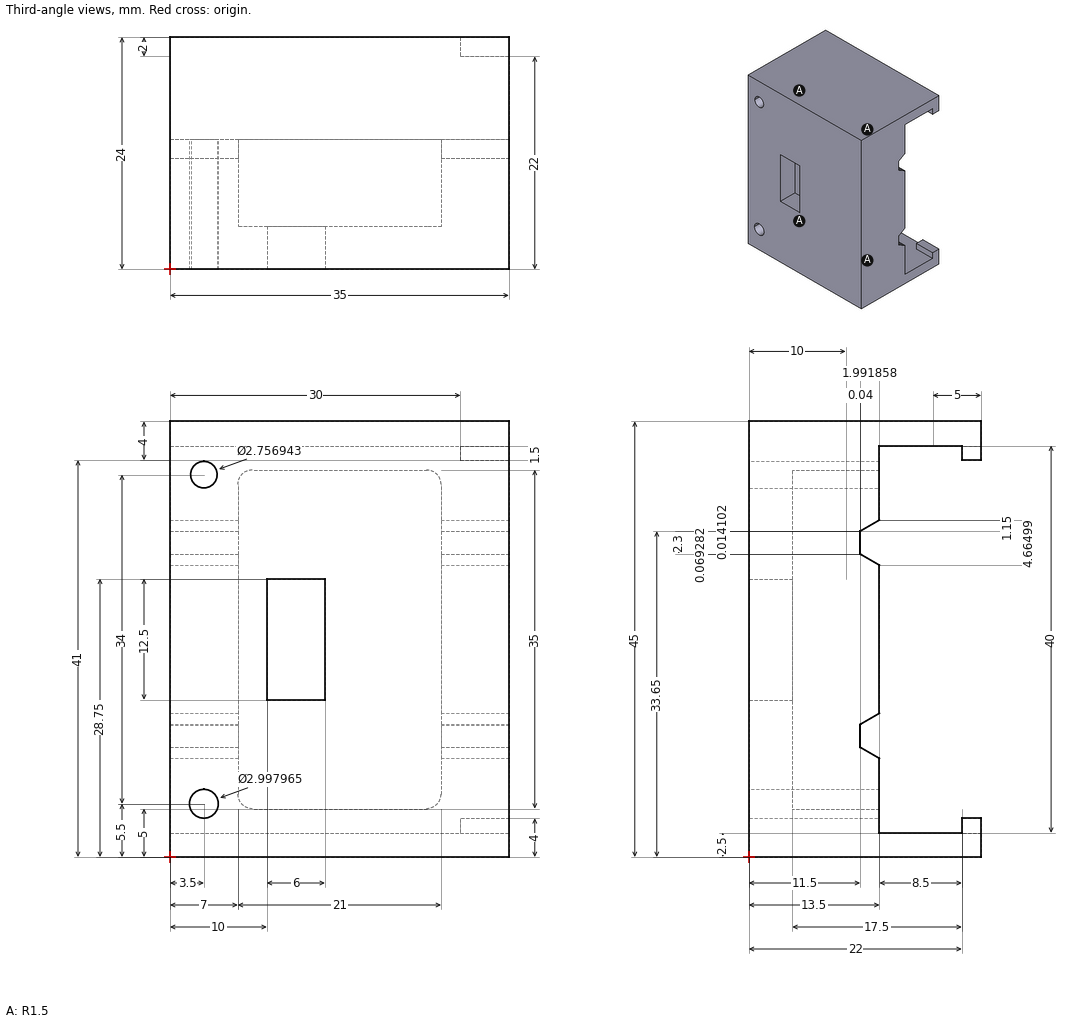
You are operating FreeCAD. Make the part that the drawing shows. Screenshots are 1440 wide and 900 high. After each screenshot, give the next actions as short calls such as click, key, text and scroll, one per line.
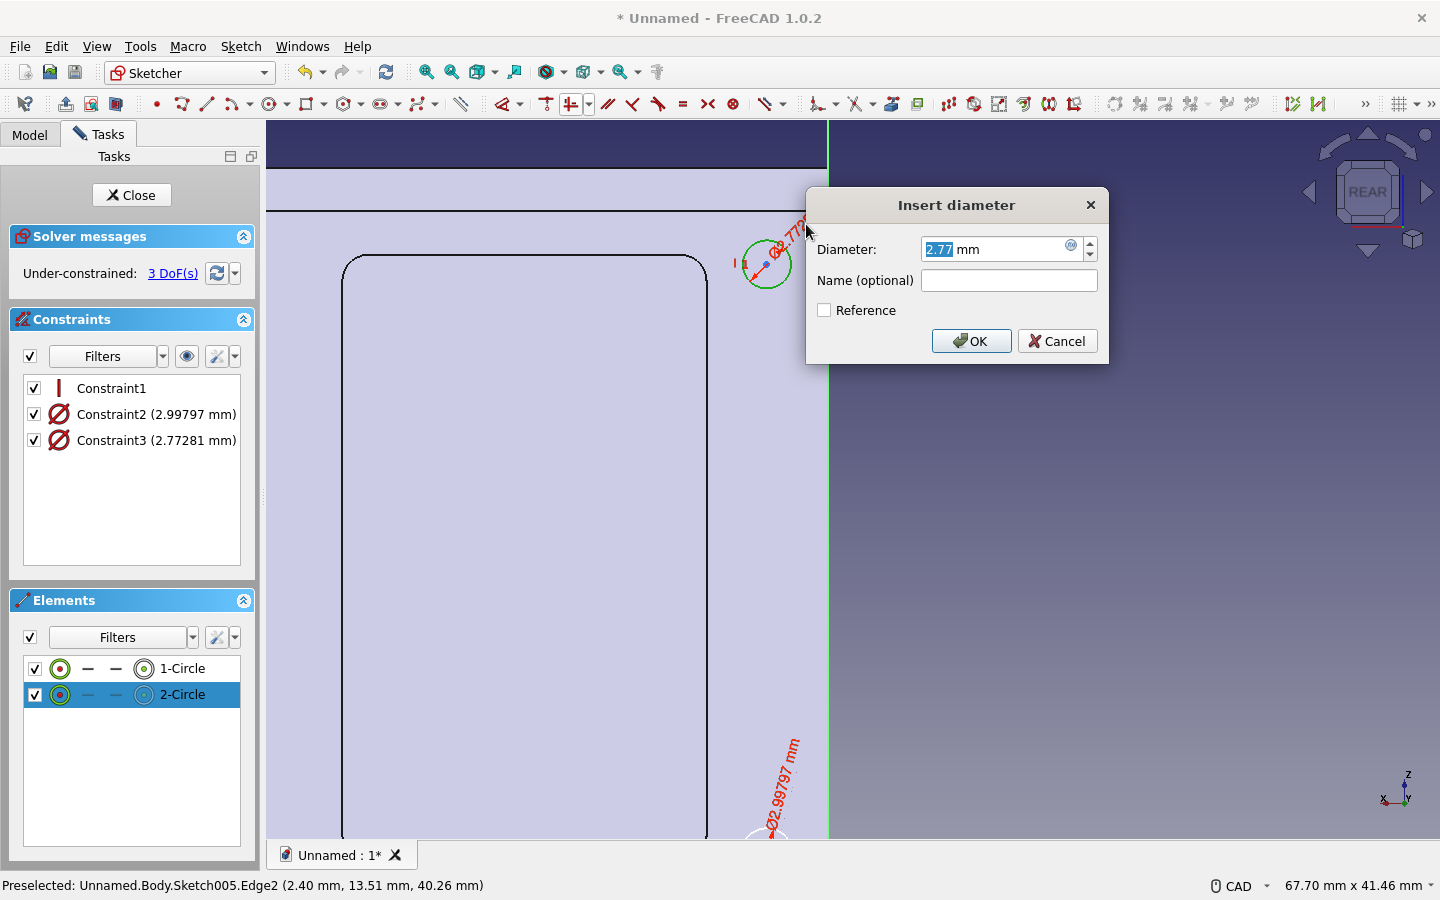
text(2.756943)
key(Return)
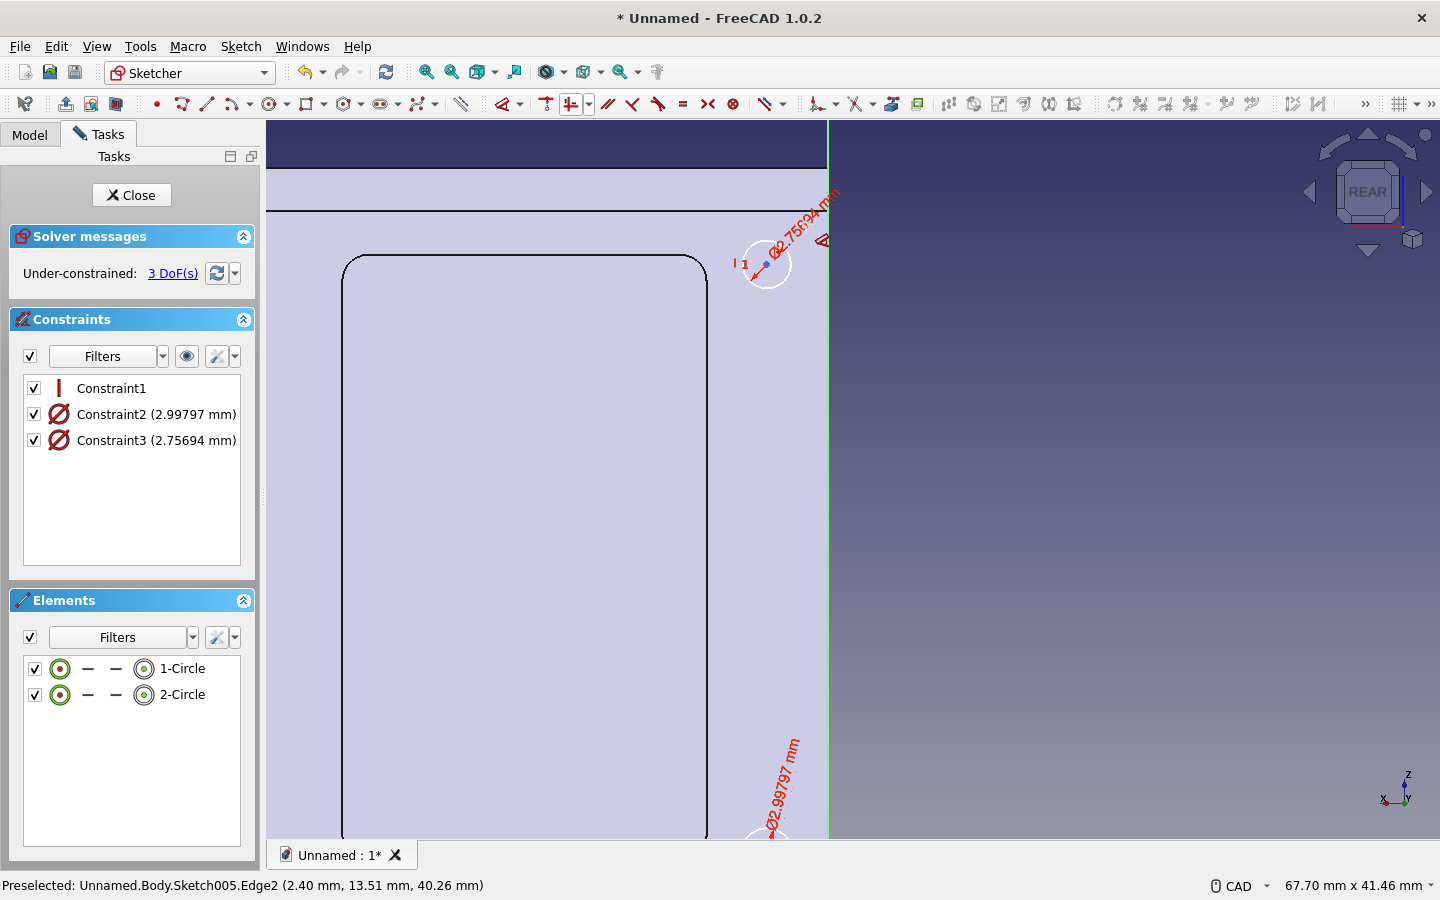
scroll(784, 247, down, 2)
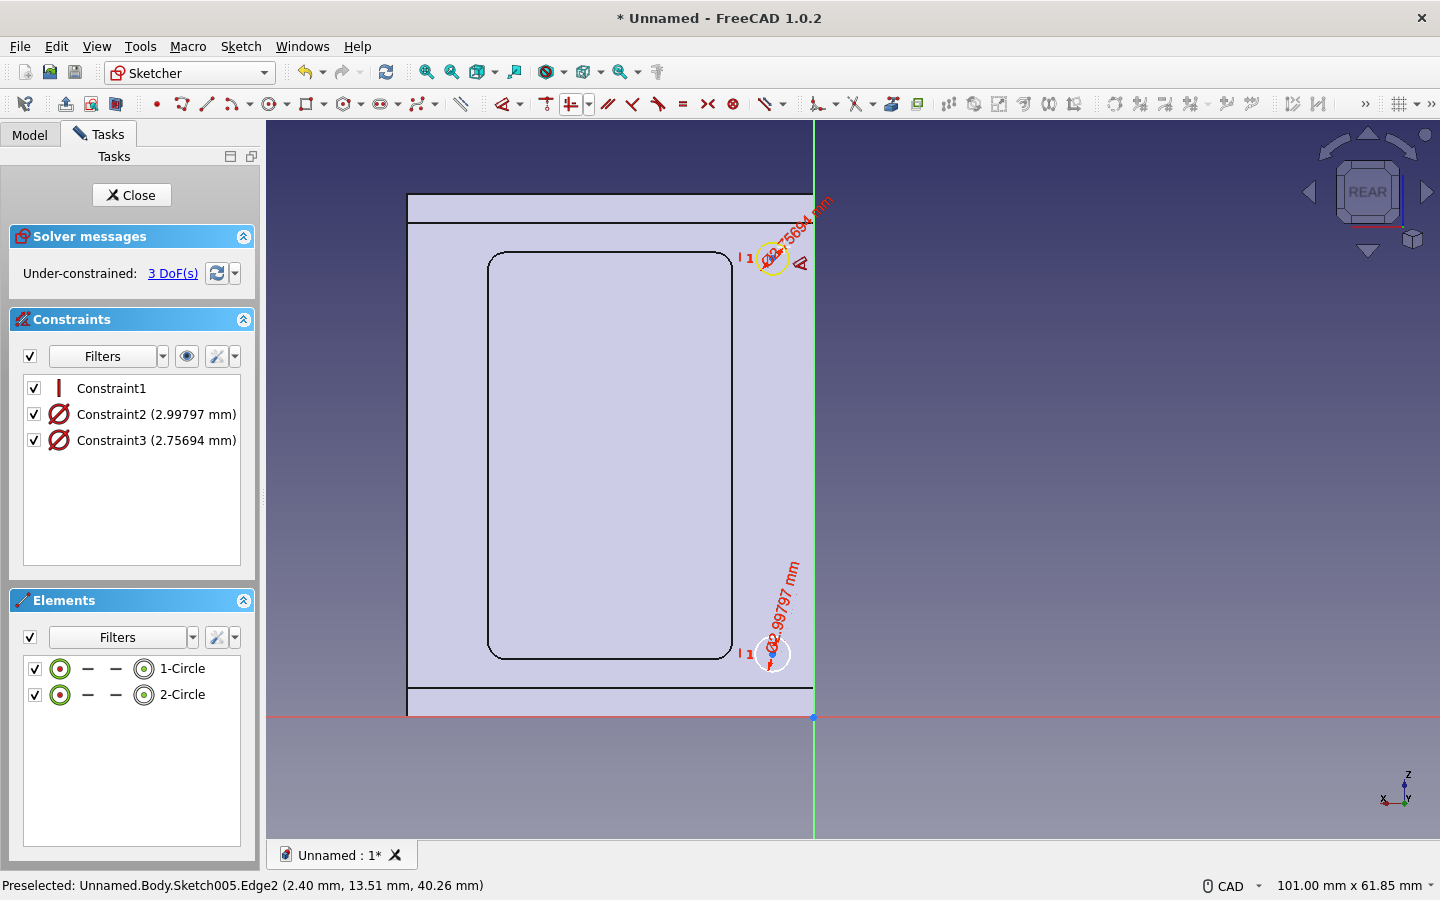
click(773, 654)
click(793, 751)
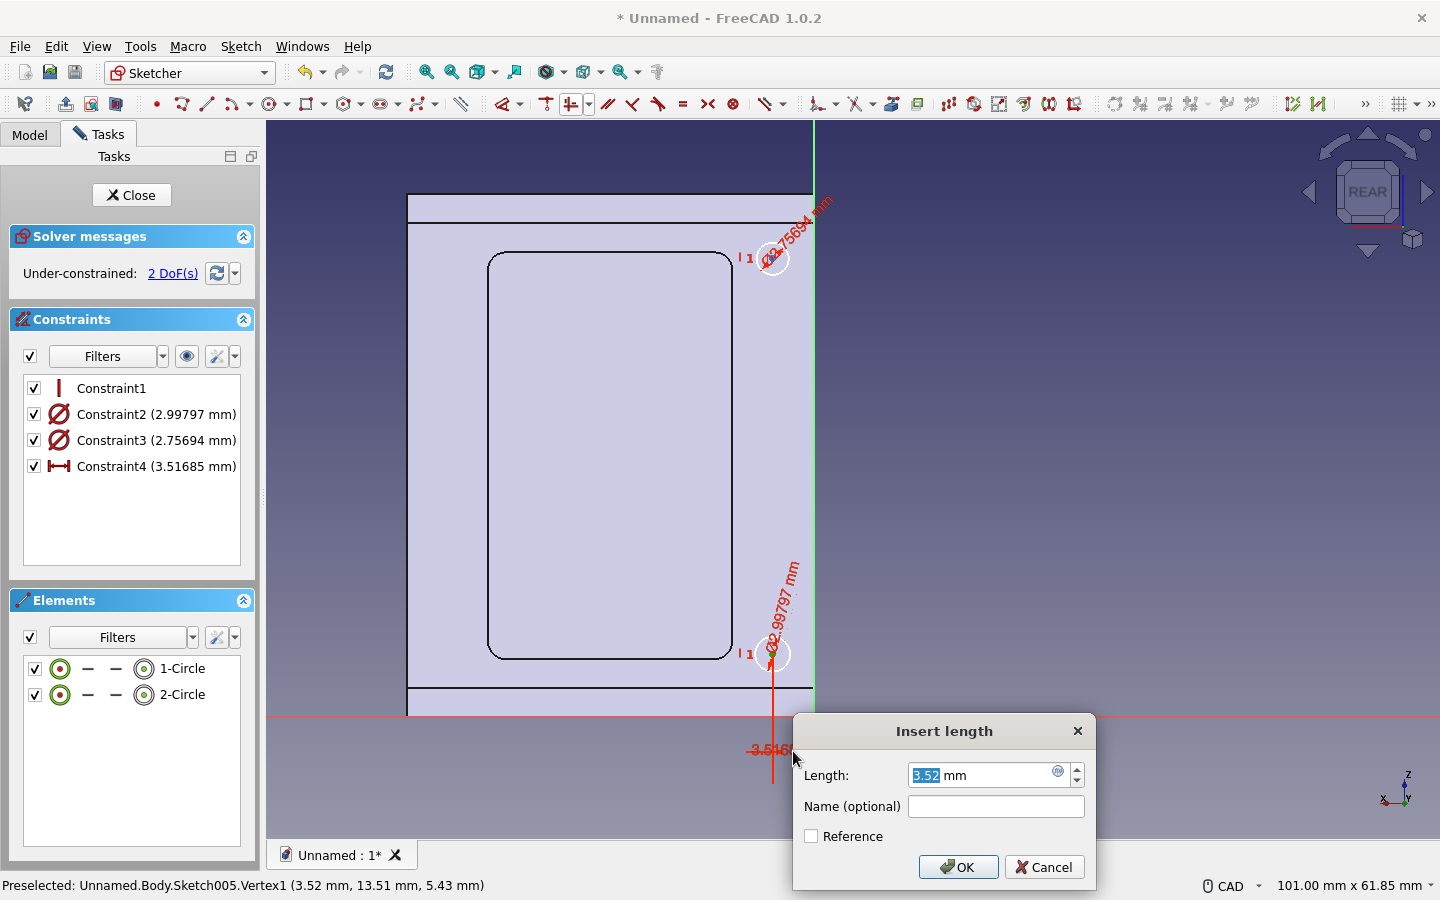
text(3.5)
key(Return)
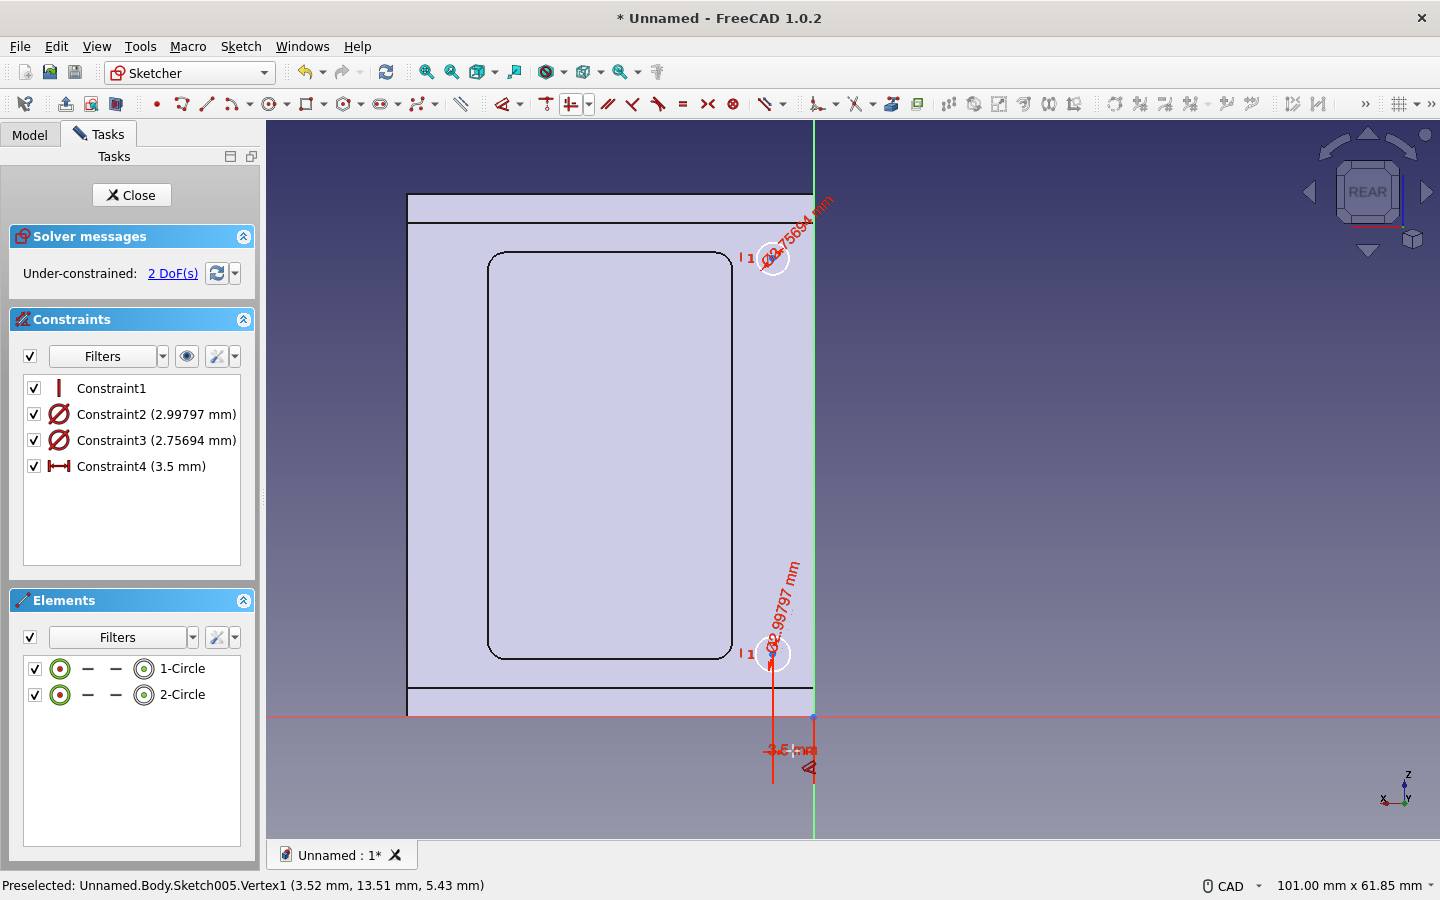
click(773, 654)
click(848, 686)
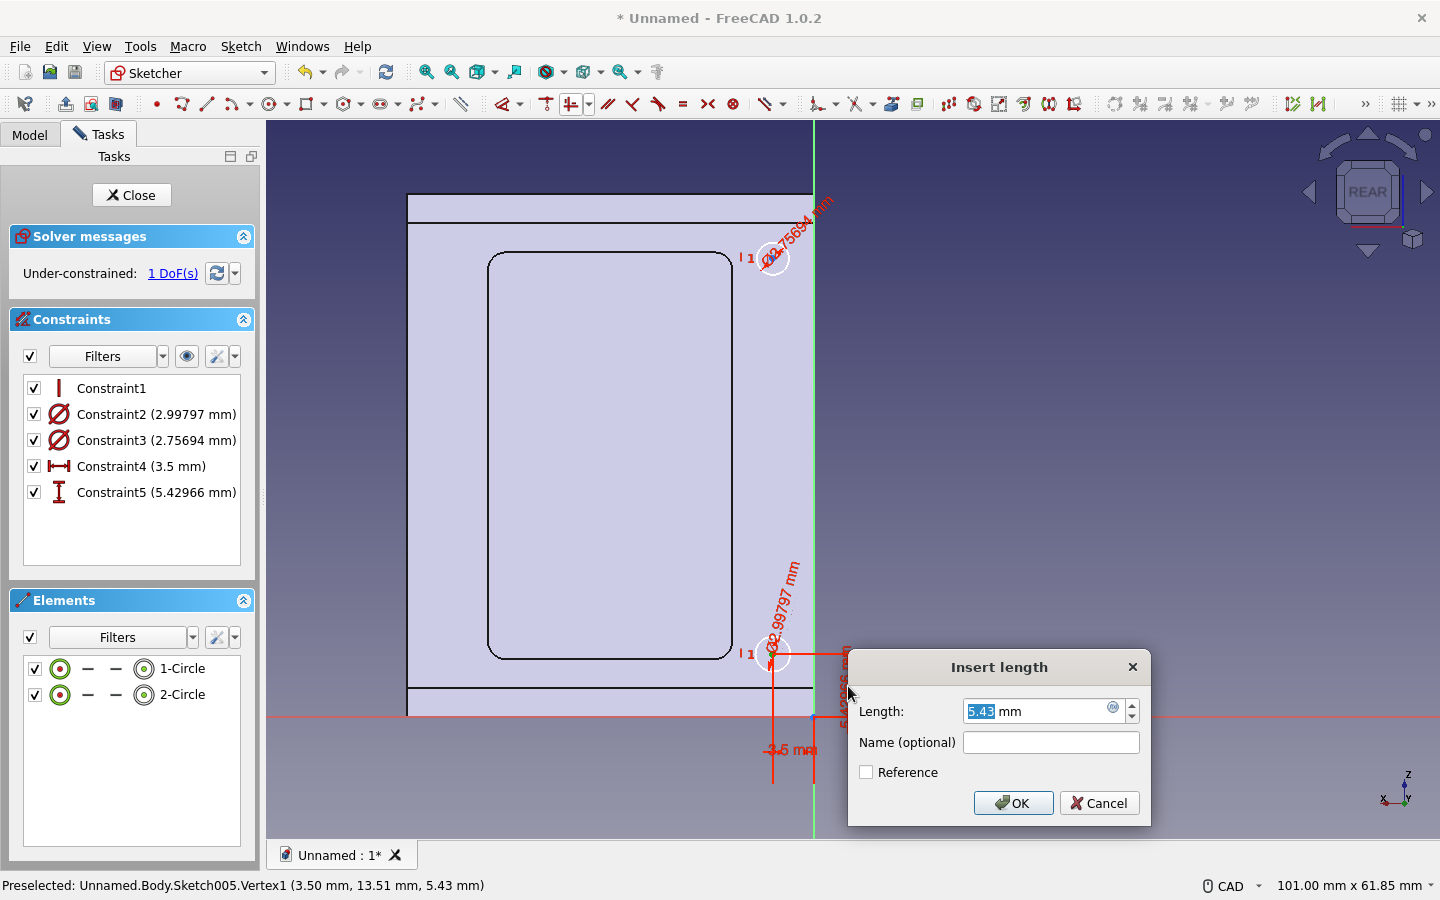
text(5.5)
key(Return)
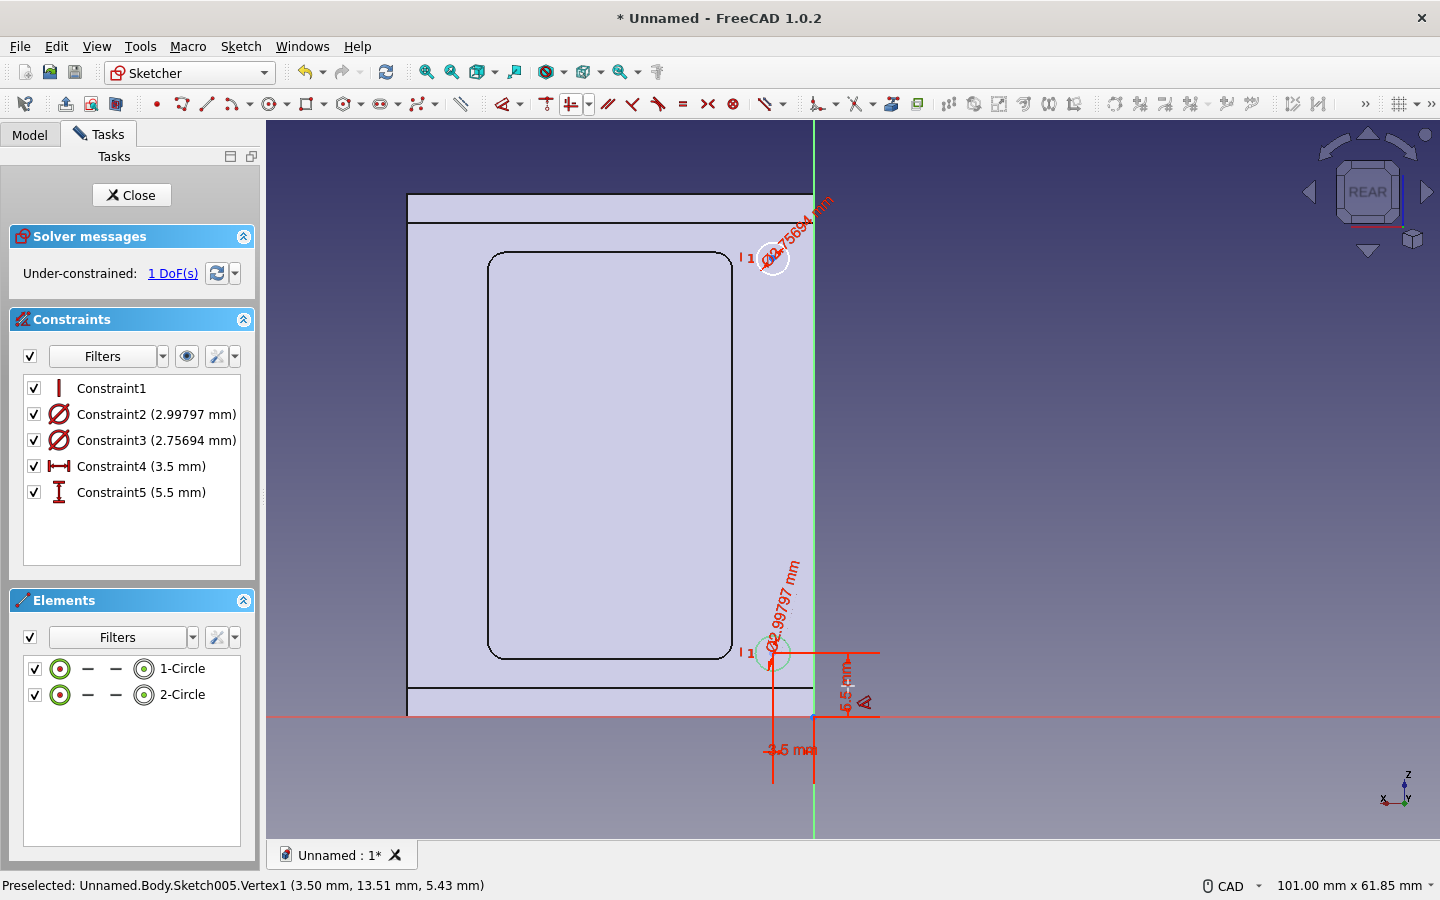
click(773, 653)